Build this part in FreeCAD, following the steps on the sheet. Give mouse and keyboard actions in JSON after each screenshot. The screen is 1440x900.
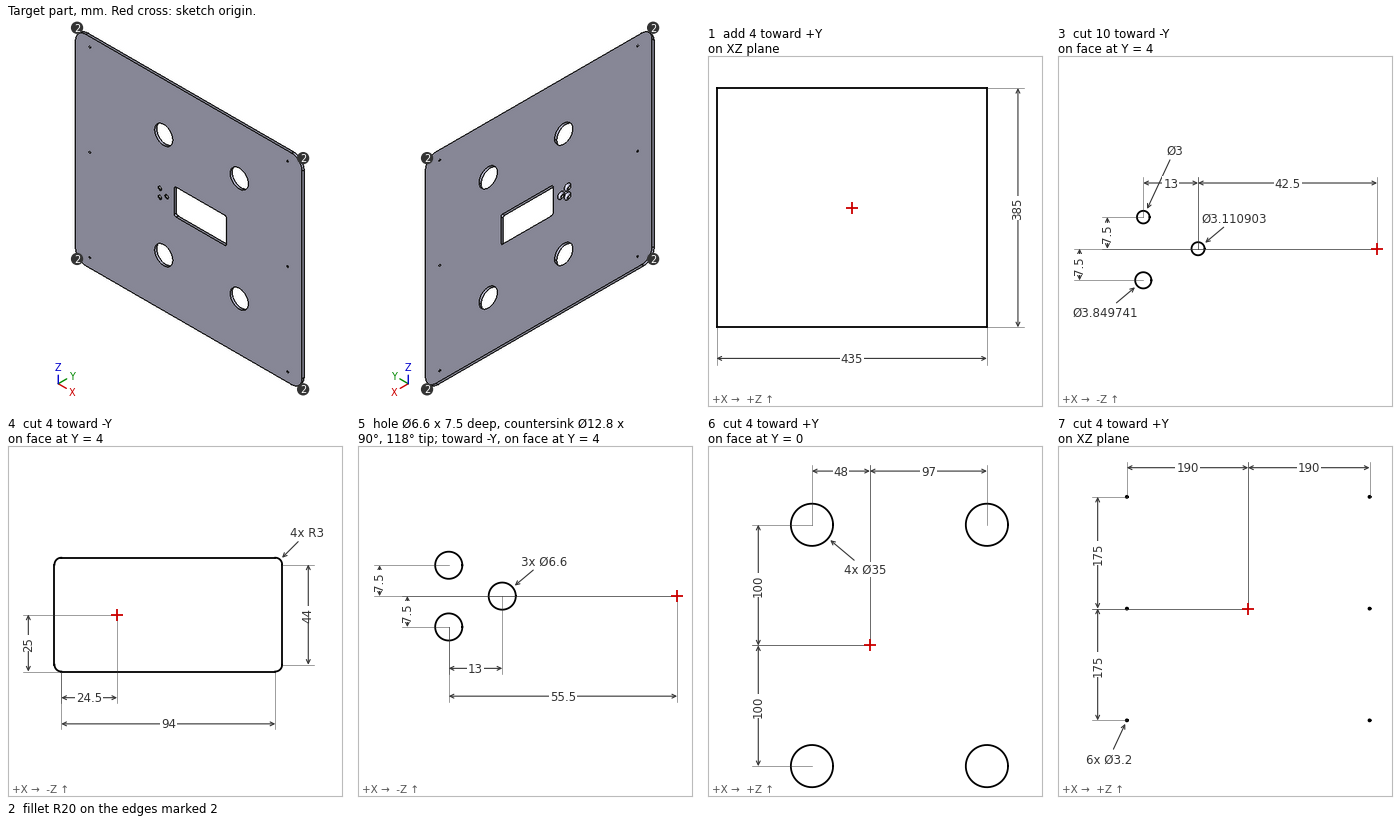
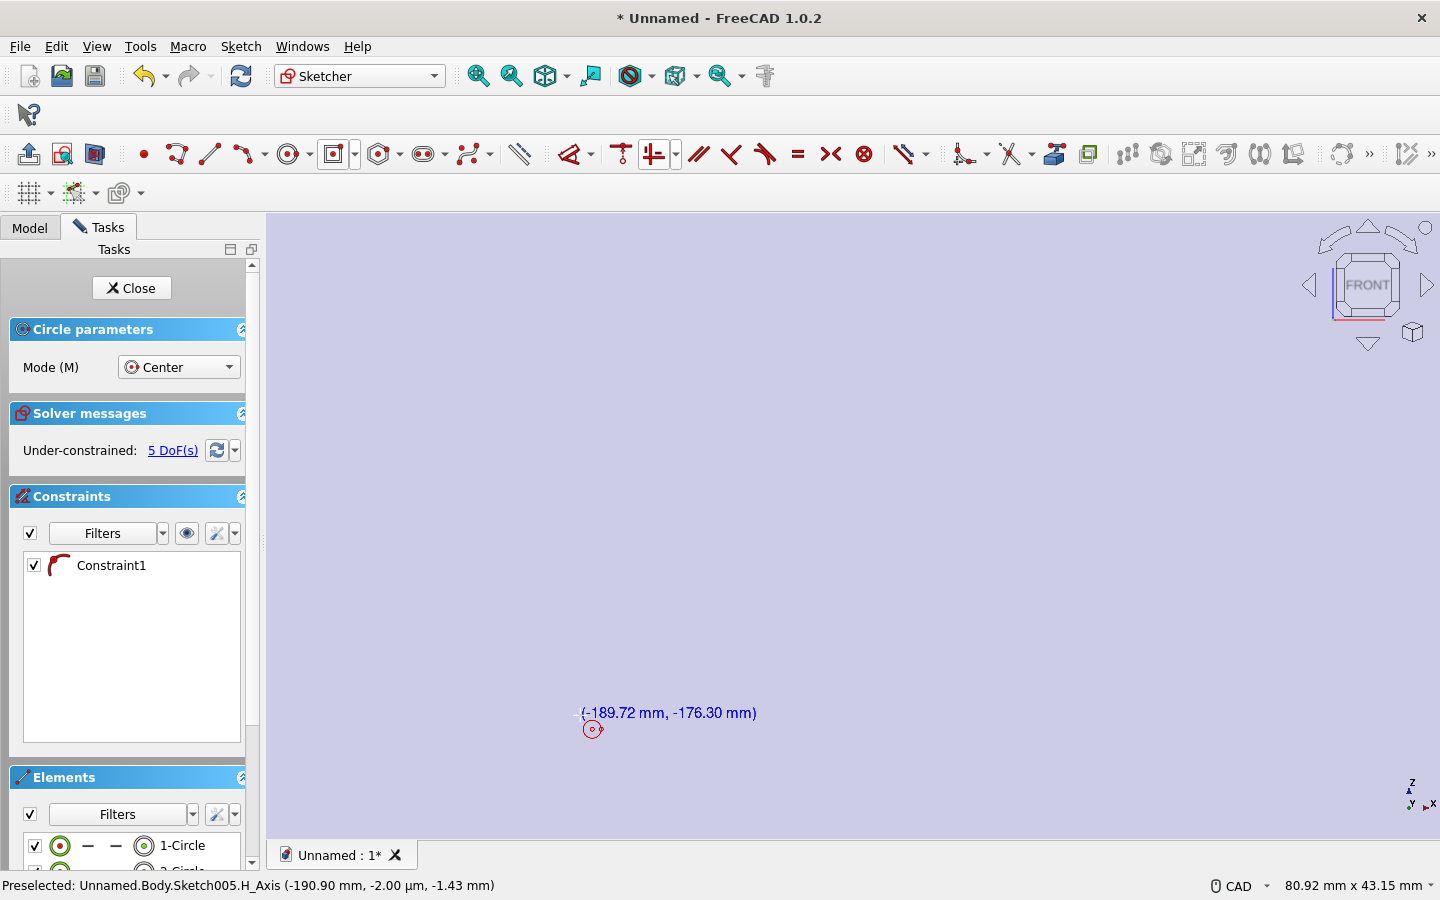
{"action": "scroll", "coordinate": [580, 716], "scroll_direction": "down", "scroll_amount": 13}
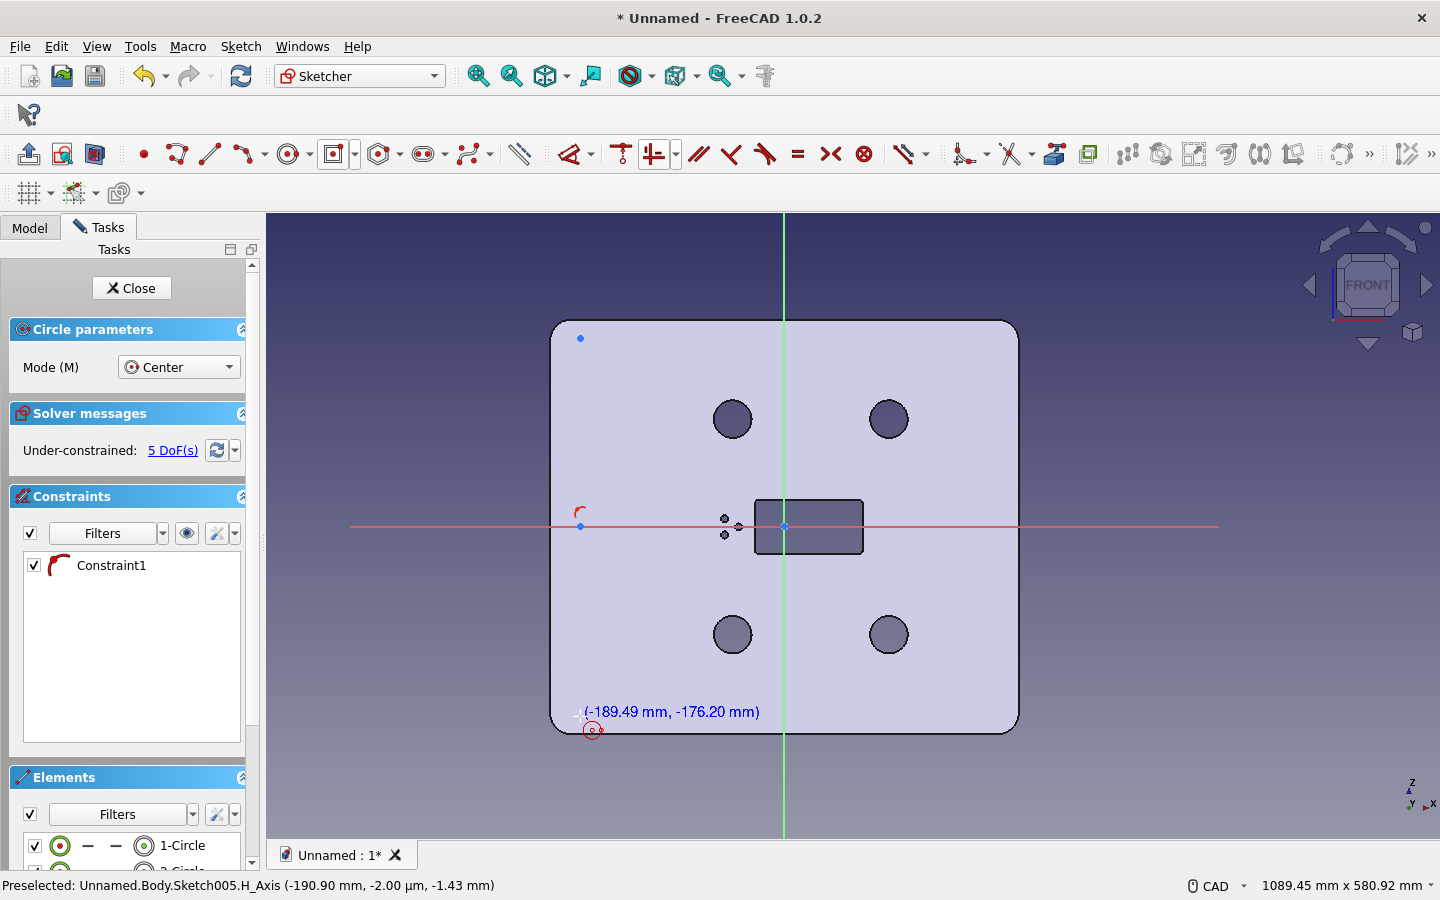
{"action": "left_click", "coordinate": [580, 716]}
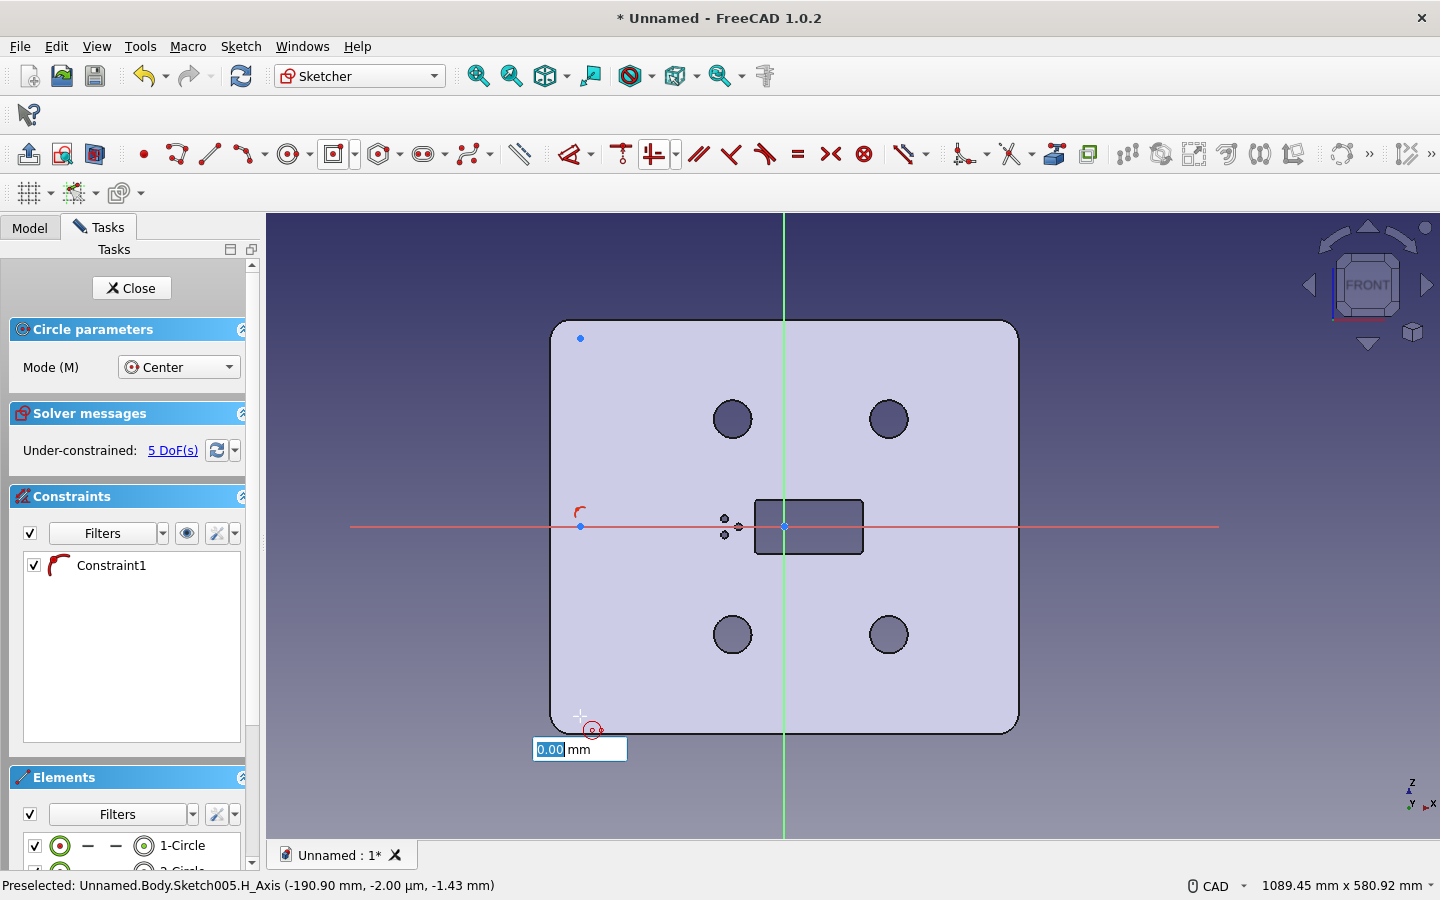
{"action": "scroll", "coordinate": [581, 714], "scroll_direction": "up", "scroll_amount": 12}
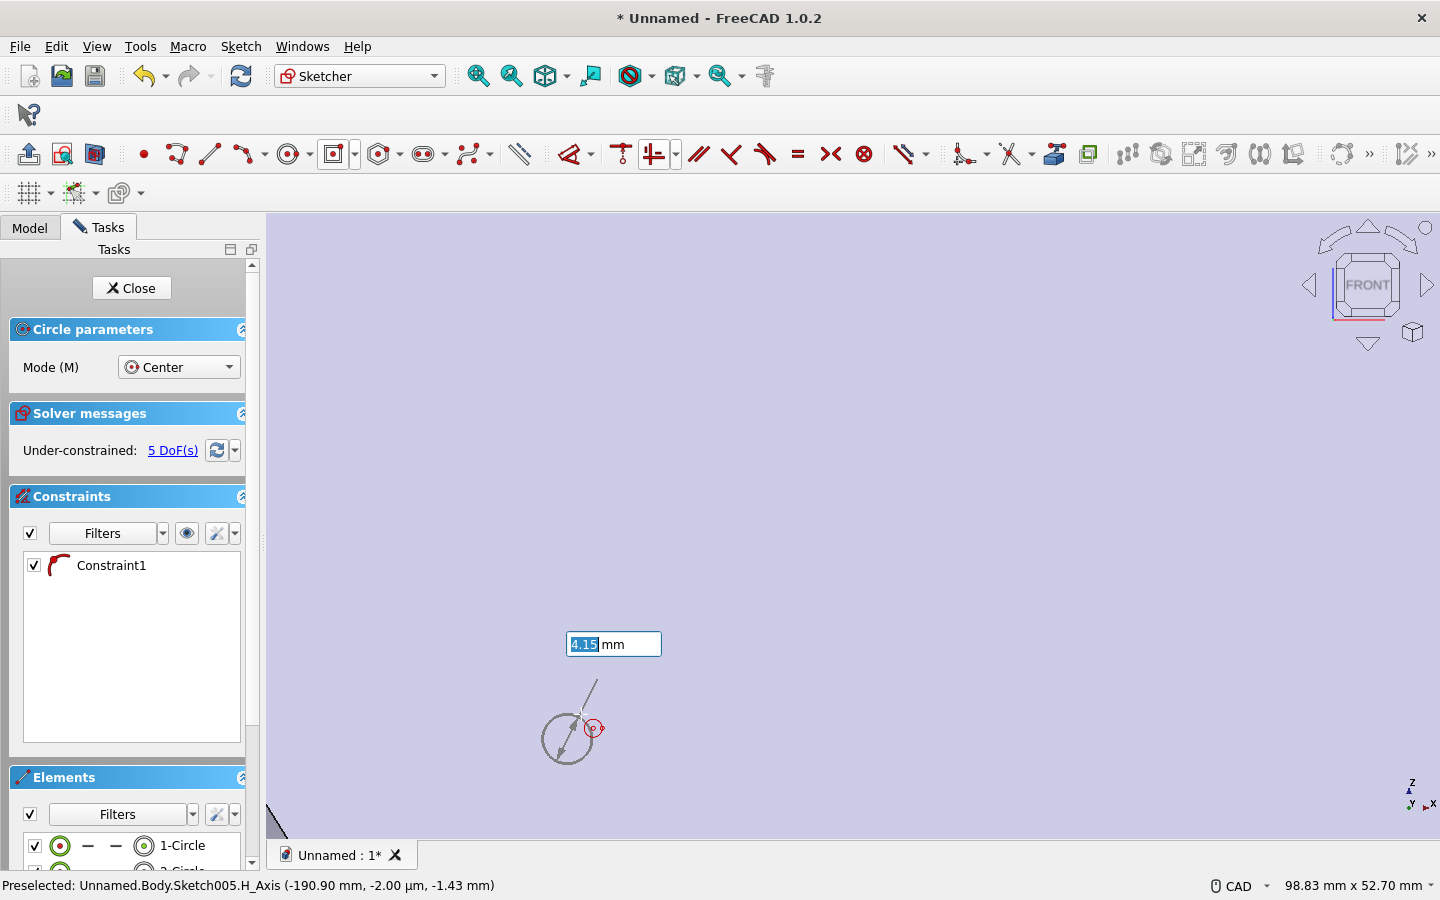
{"action": "left_click", "coordinate": [577, 709]}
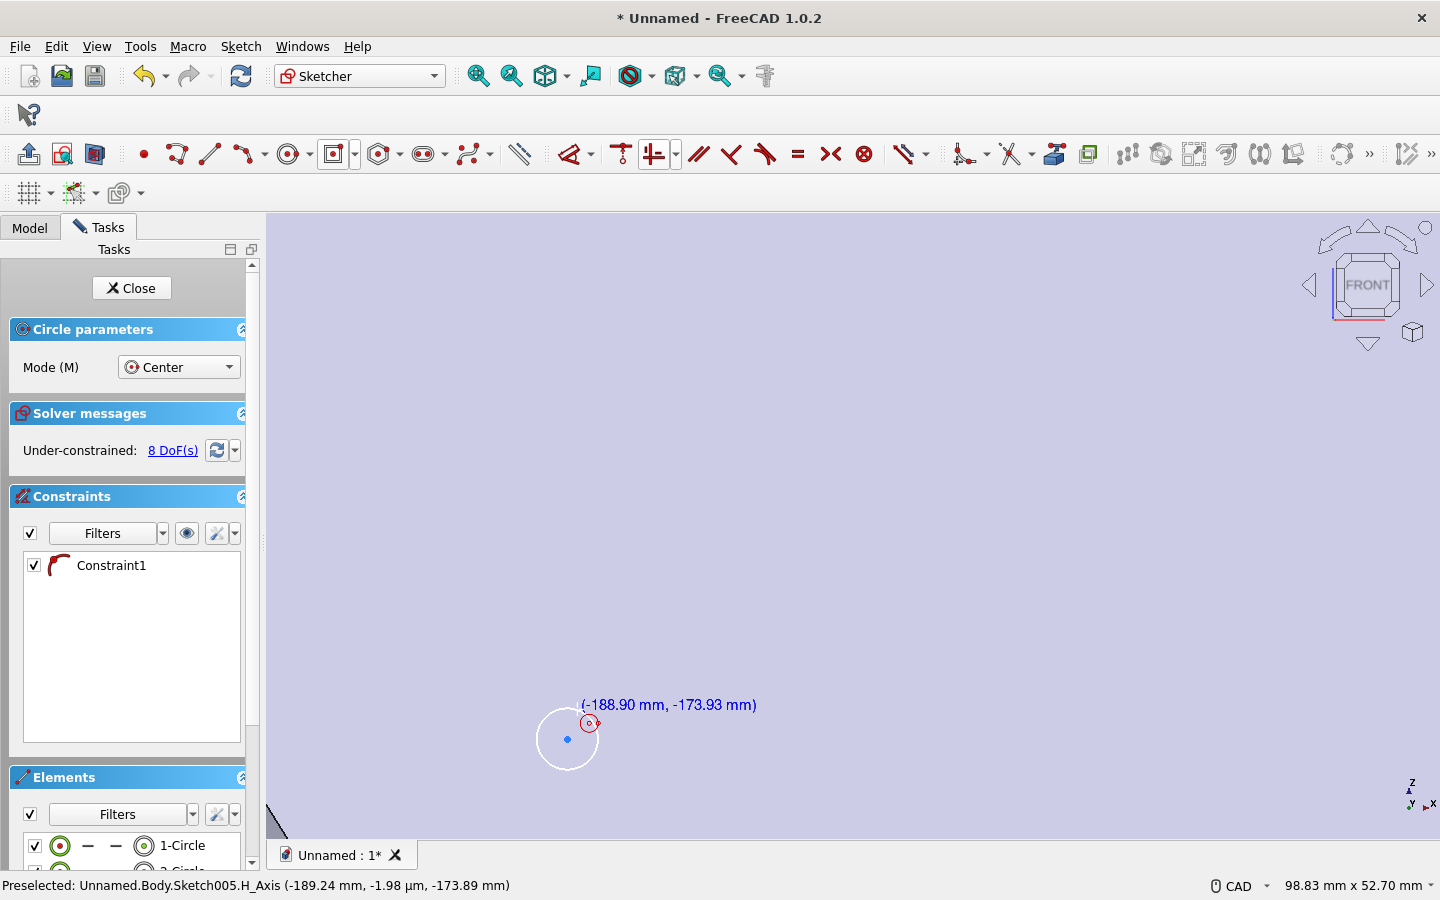
{"action": "scroll", "coordinate": [581, 714], "scroll_direction": "down", "scroll_amount": 12}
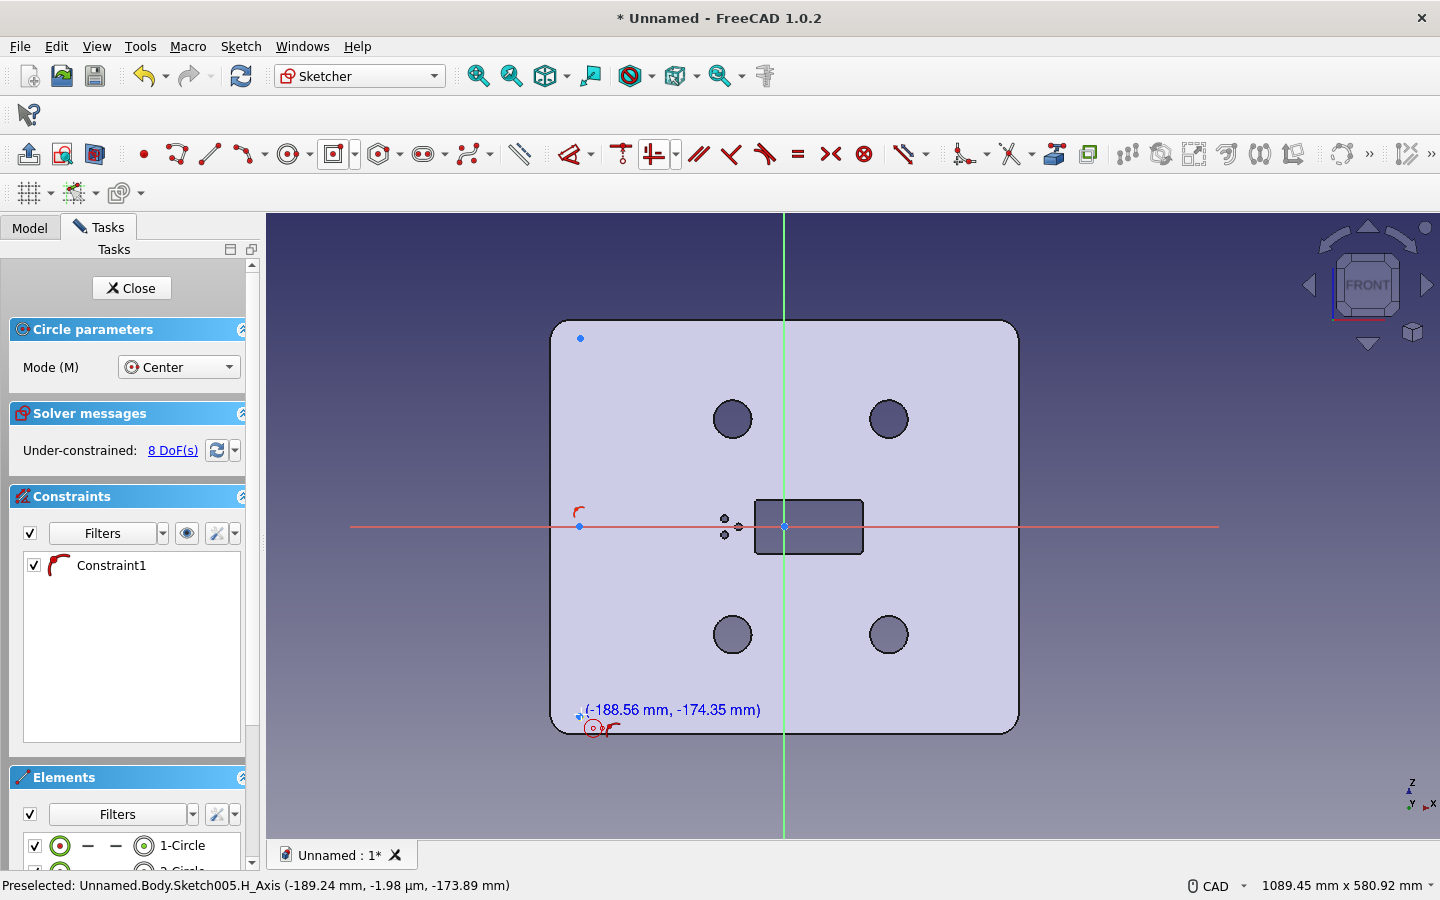
{"action": "scroll", "coordinate": [989, 338], "scroll_direction": "up", "scroll_amount": 13}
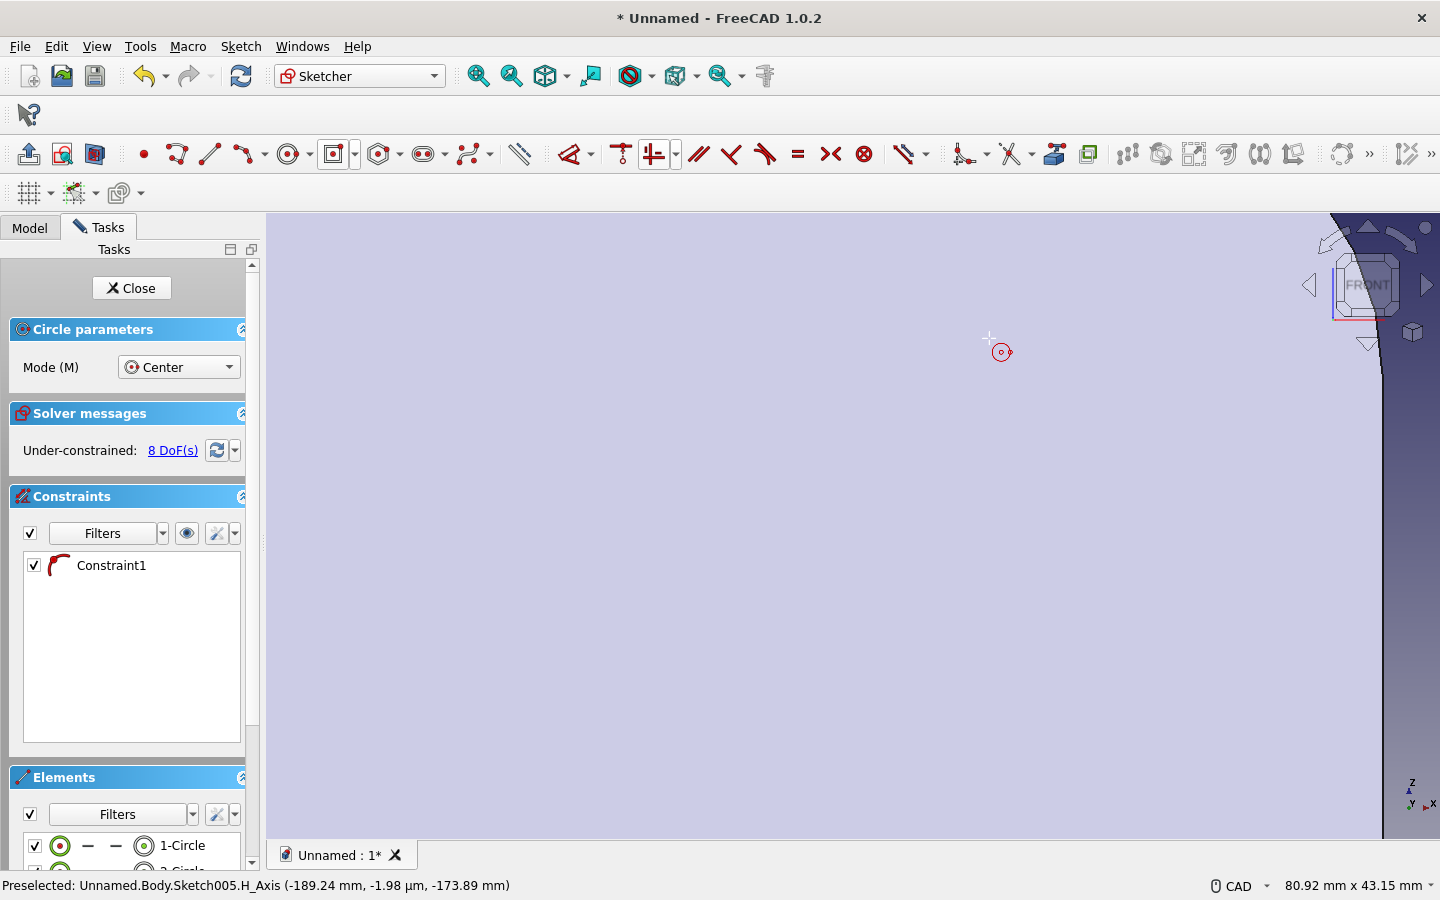
{"action": "scroll", "coordinate": [990, 337], "scroll_direction": "down", "scroll_amount": 13}